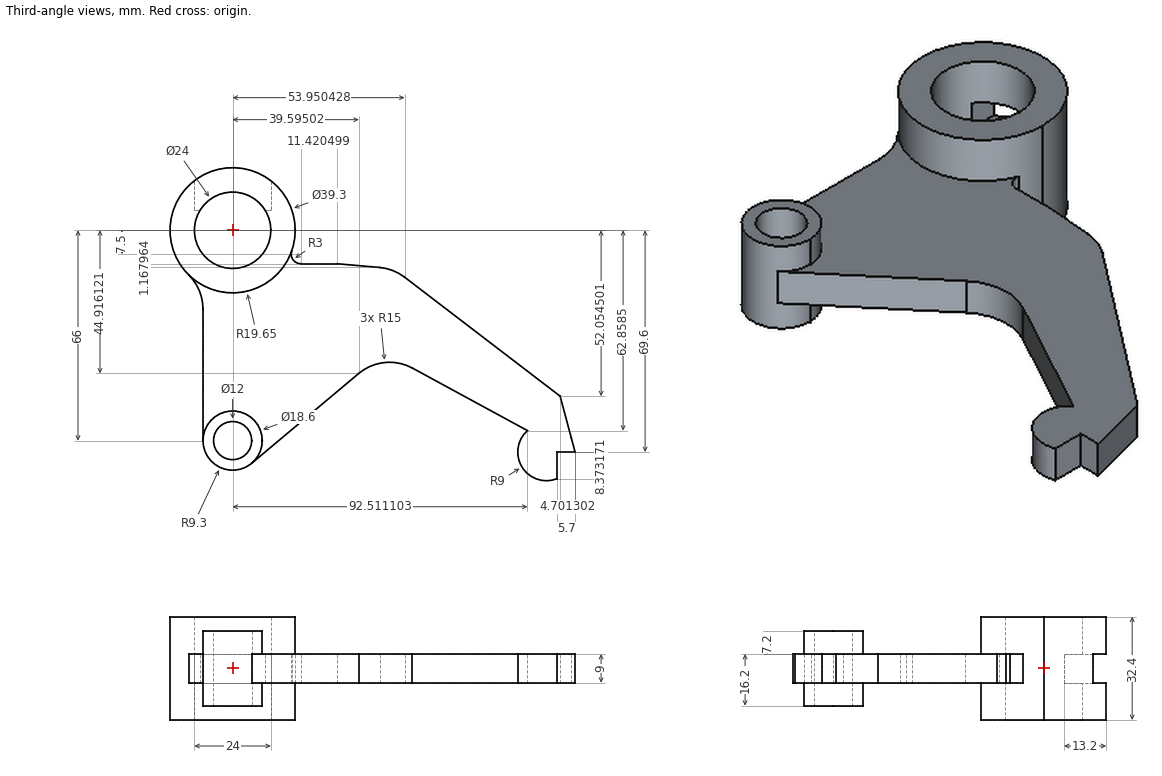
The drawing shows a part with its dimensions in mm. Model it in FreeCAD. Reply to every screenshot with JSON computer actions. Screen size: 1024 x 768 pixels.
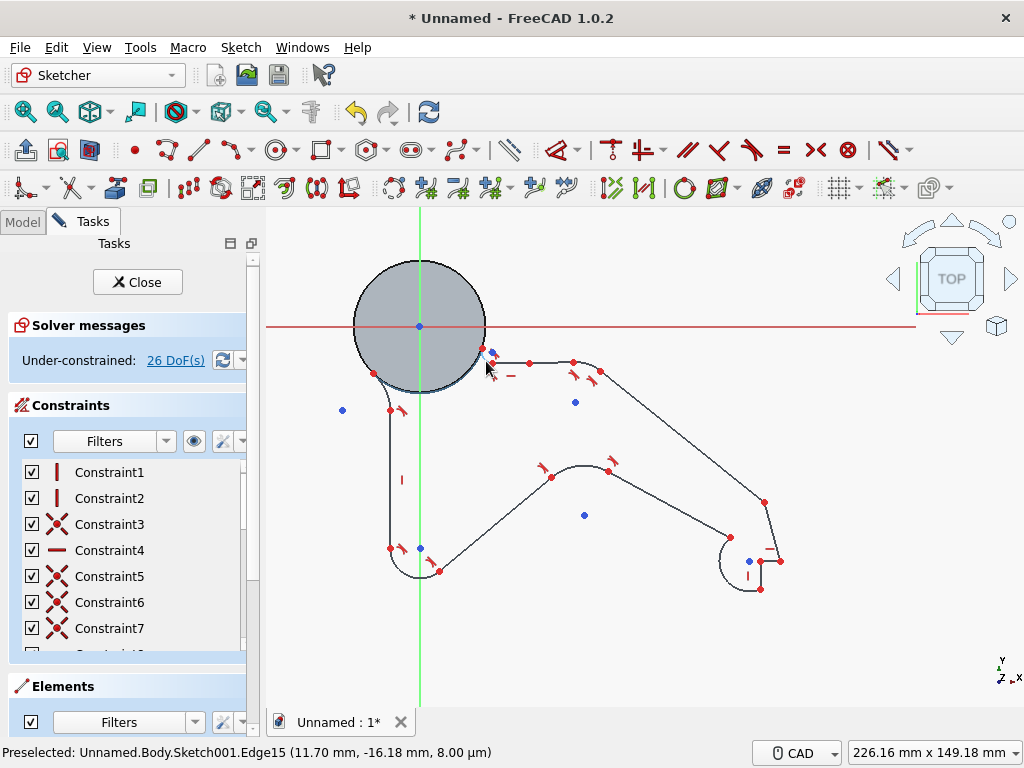
{"action": "left_click", "coordinate": [389, 398]}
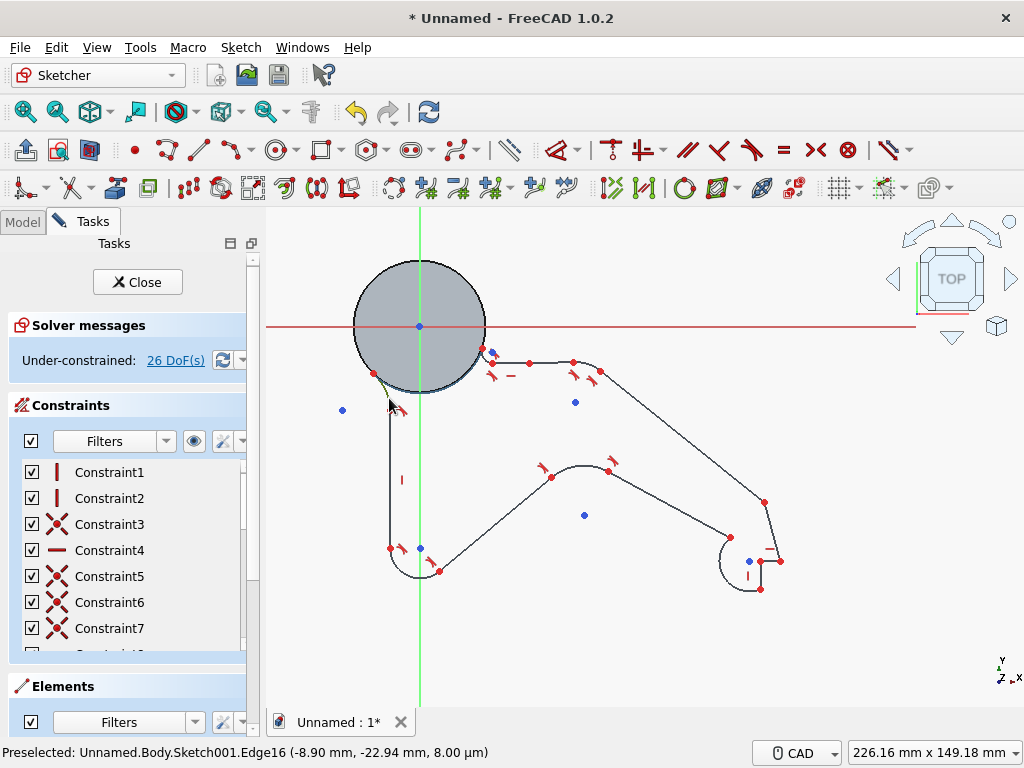
{"action": "key", "text": "t"}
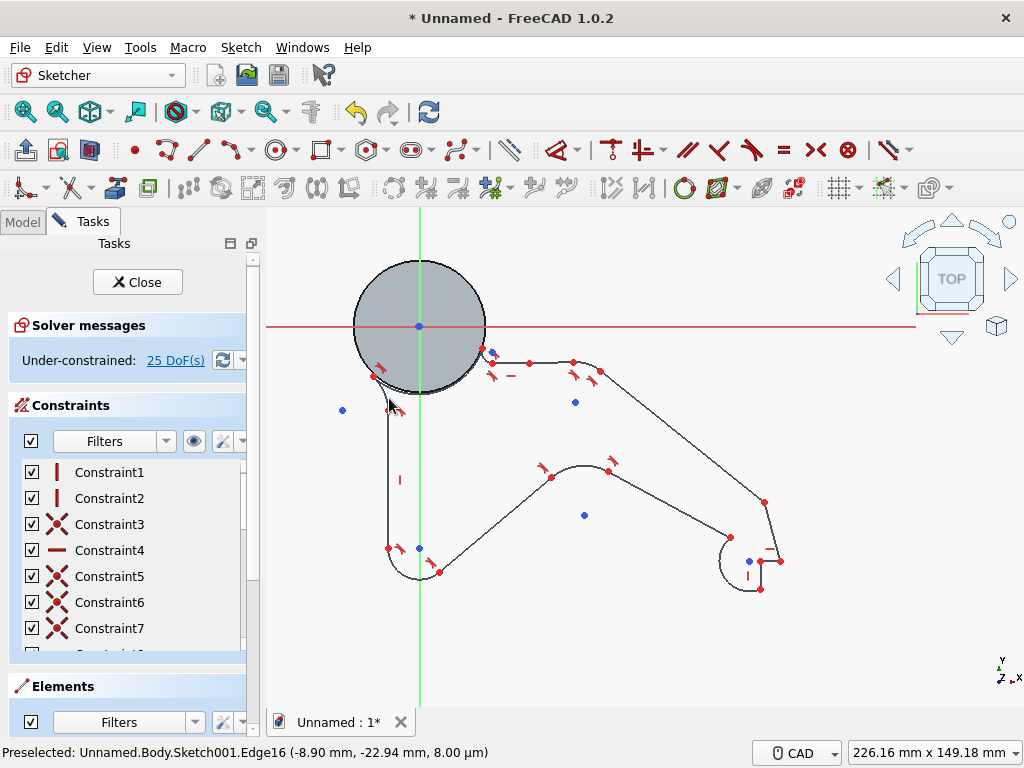
{"action": "scroll", "coordinate": [419, 327], "scroll_direction": "up", "scroll_amount": 7}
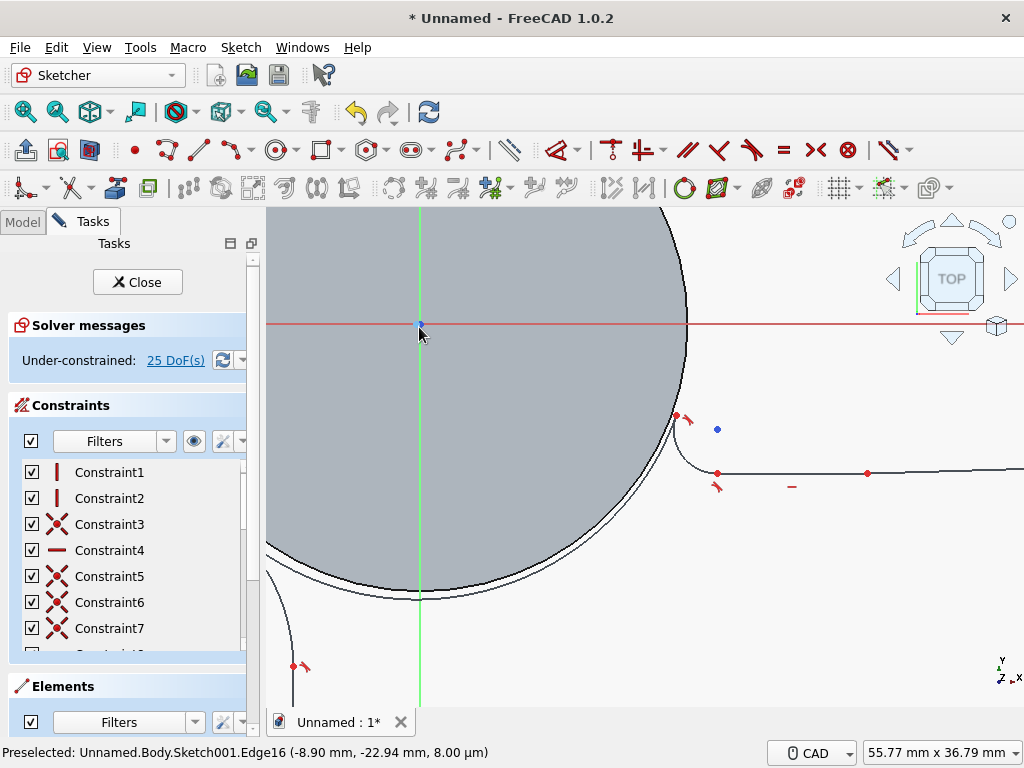
{"action": "left_click_drag", "start_coordinate": [407, 314], "coordinate": [430, 334]}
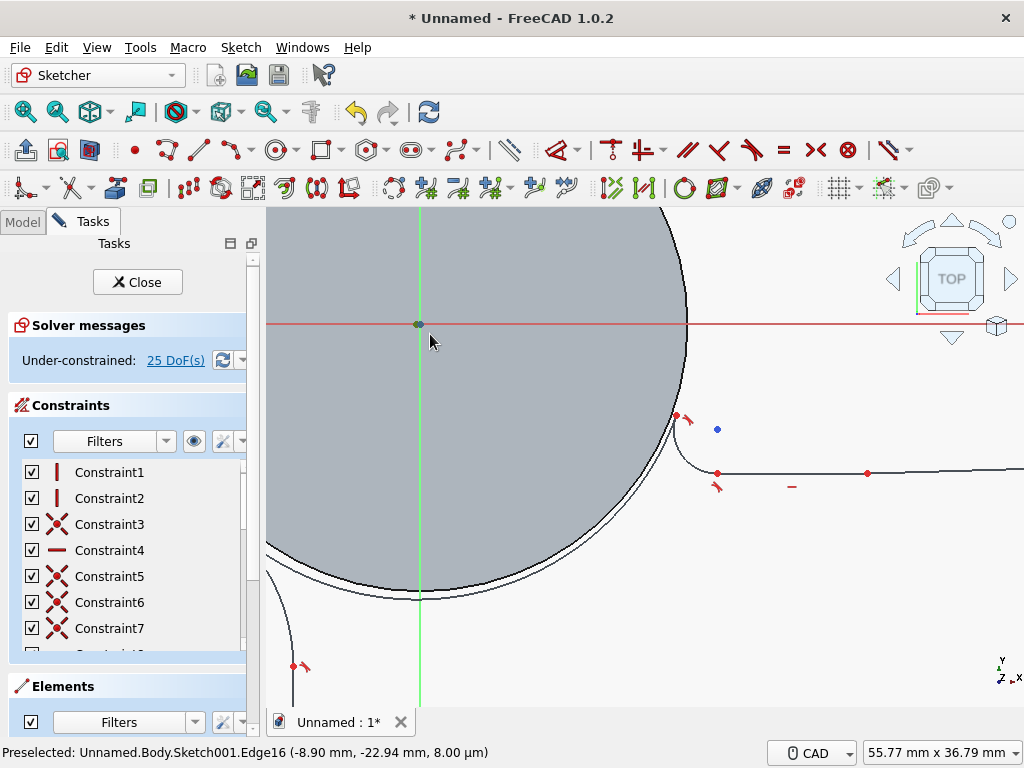
{"action": "key", "text": "c"}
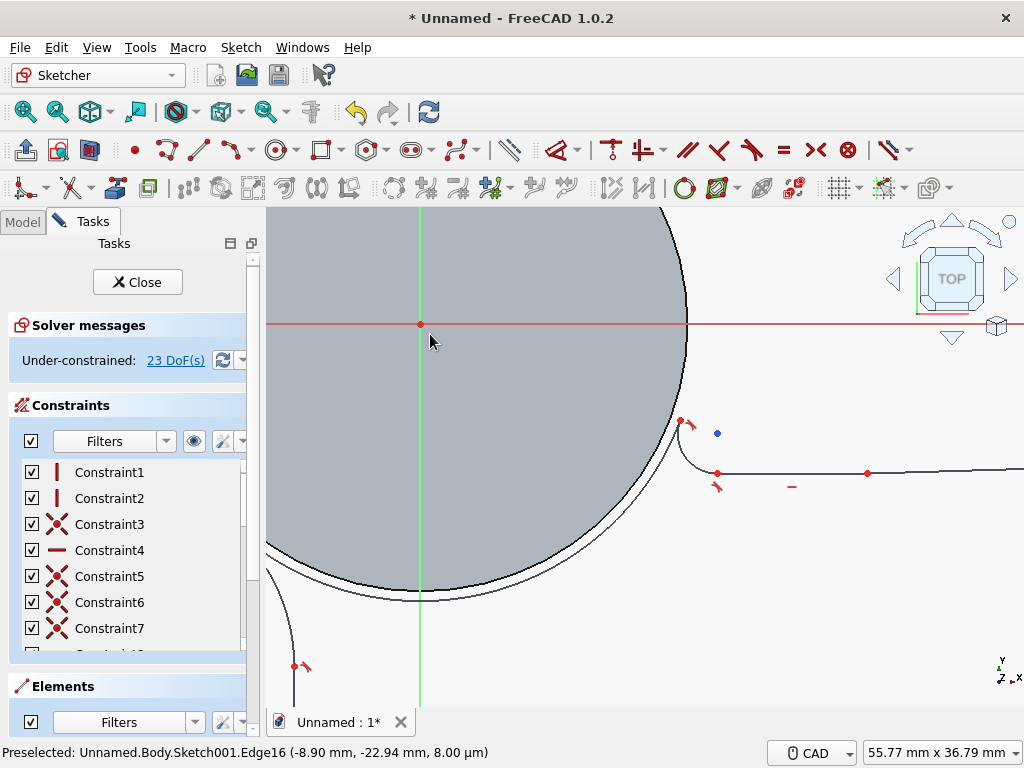
{"action": "scroll", "coordinate": [419, 327], "scroll_direction": "down", "scroll_amount": 7}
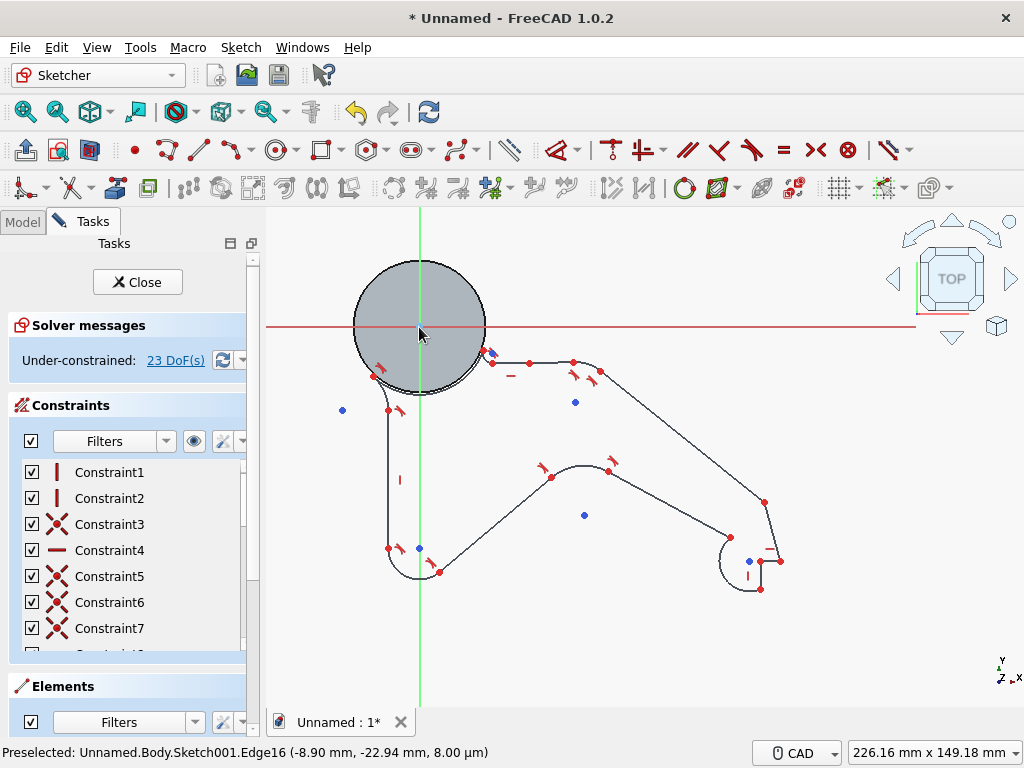
{"action": "left_click", "coordinate": [591, 466]}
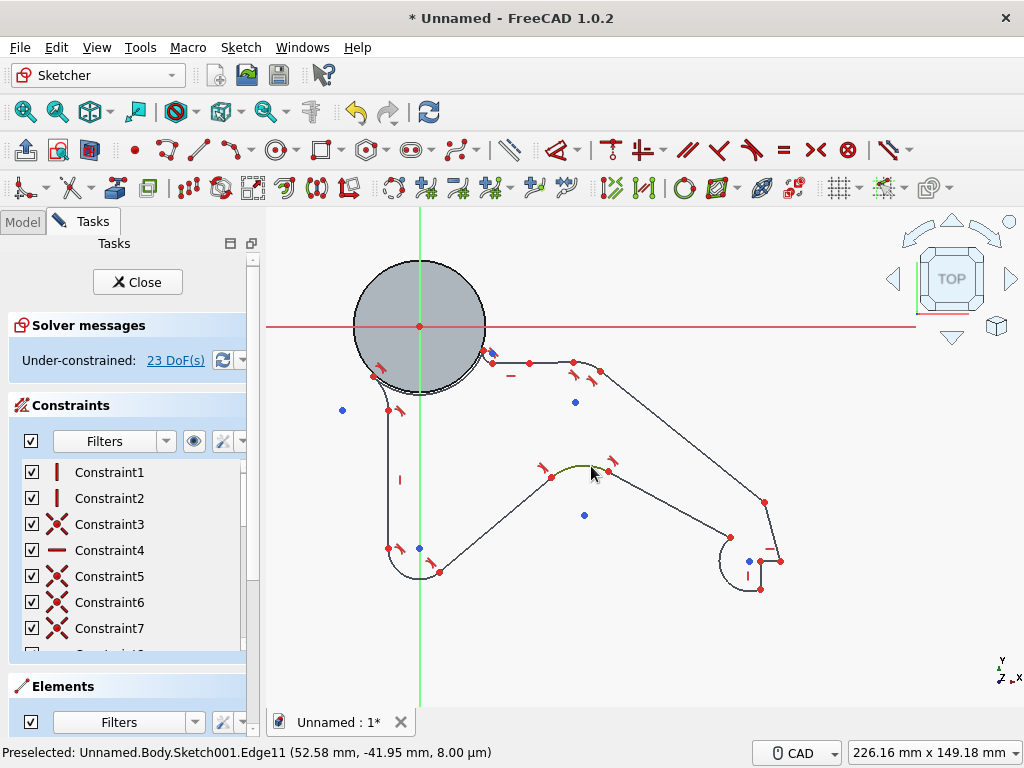
{"action": "left_click", "coordinate": [588, 364]}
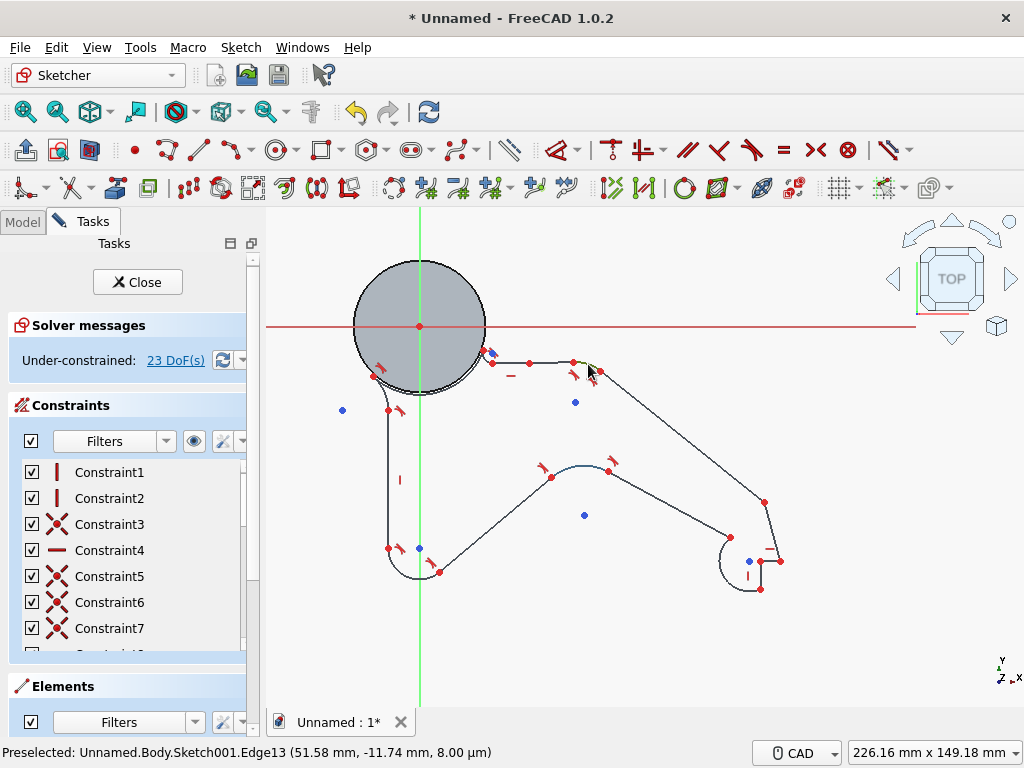
{"action": "left_click", "coordinate": [387, 400]}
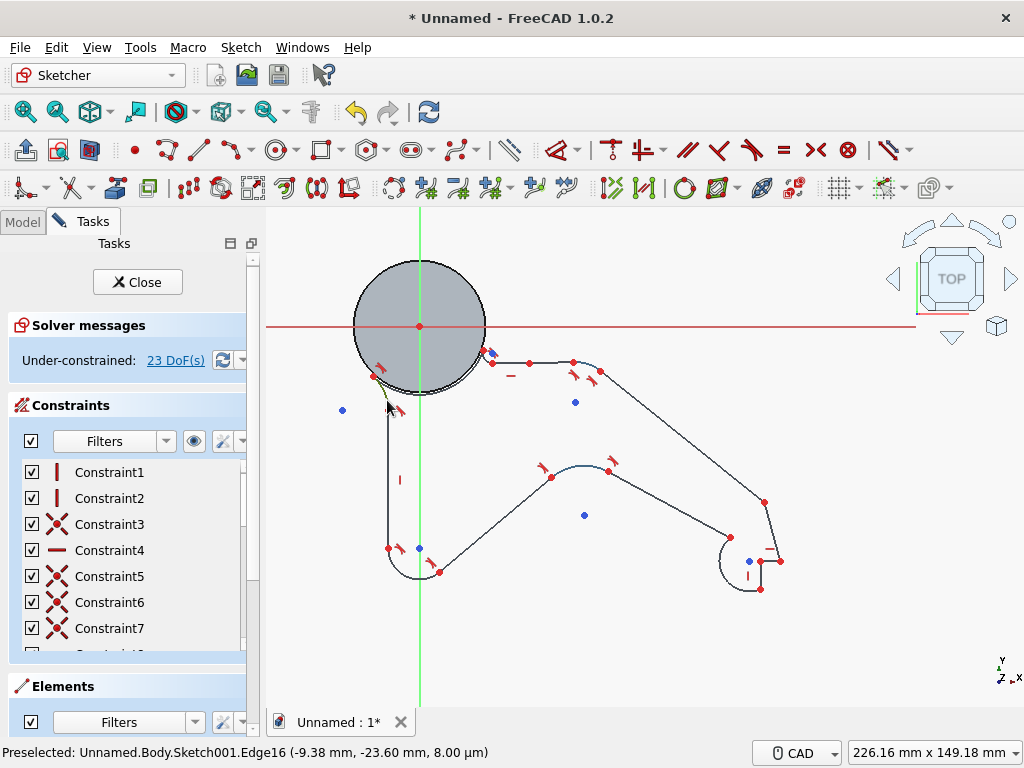
{"action": "key", "text": "e"}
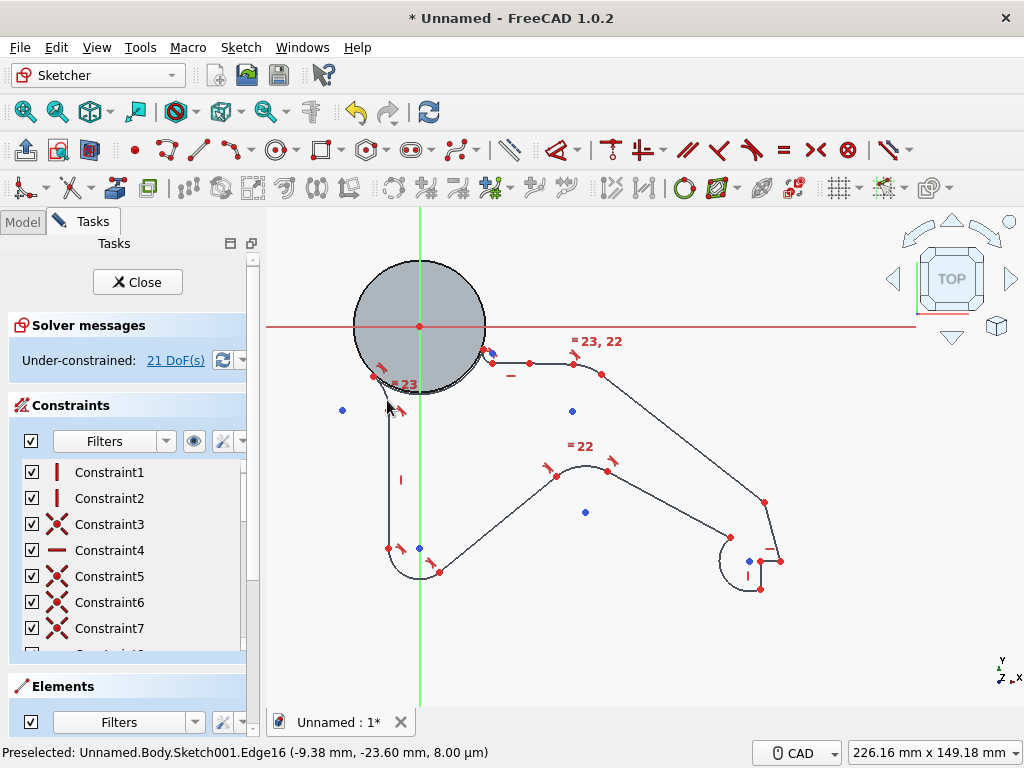
{"action": "left_click", "coordinate": [420, 548]}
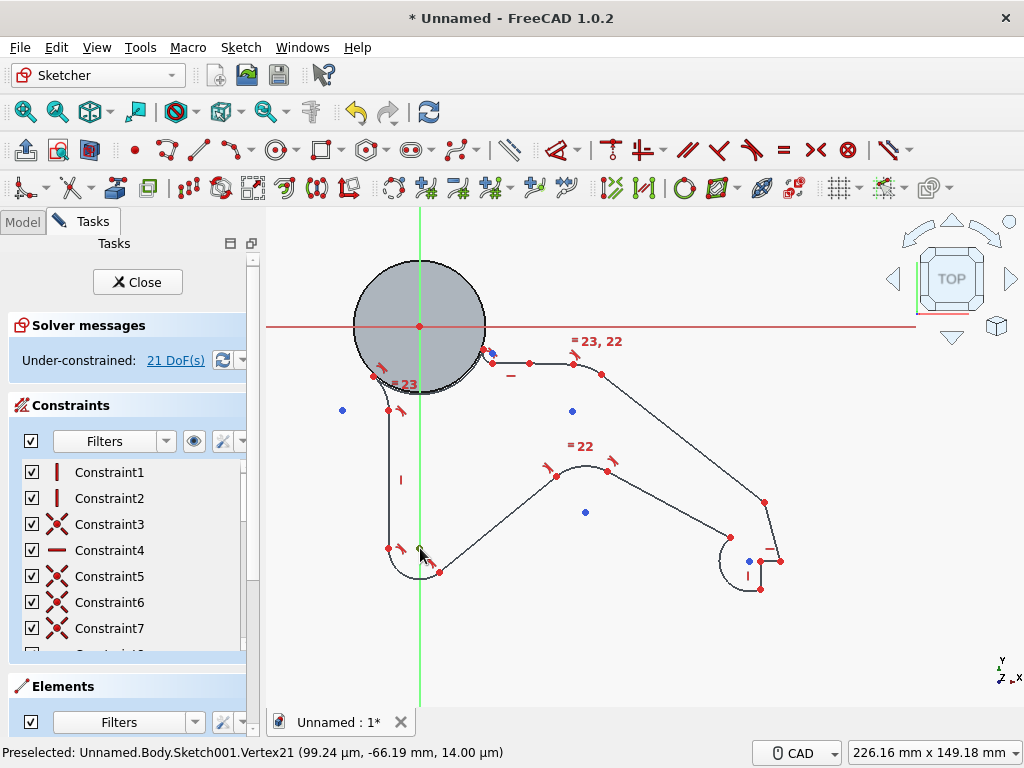
{"action": "left_click", "coordinate": [420, 647]}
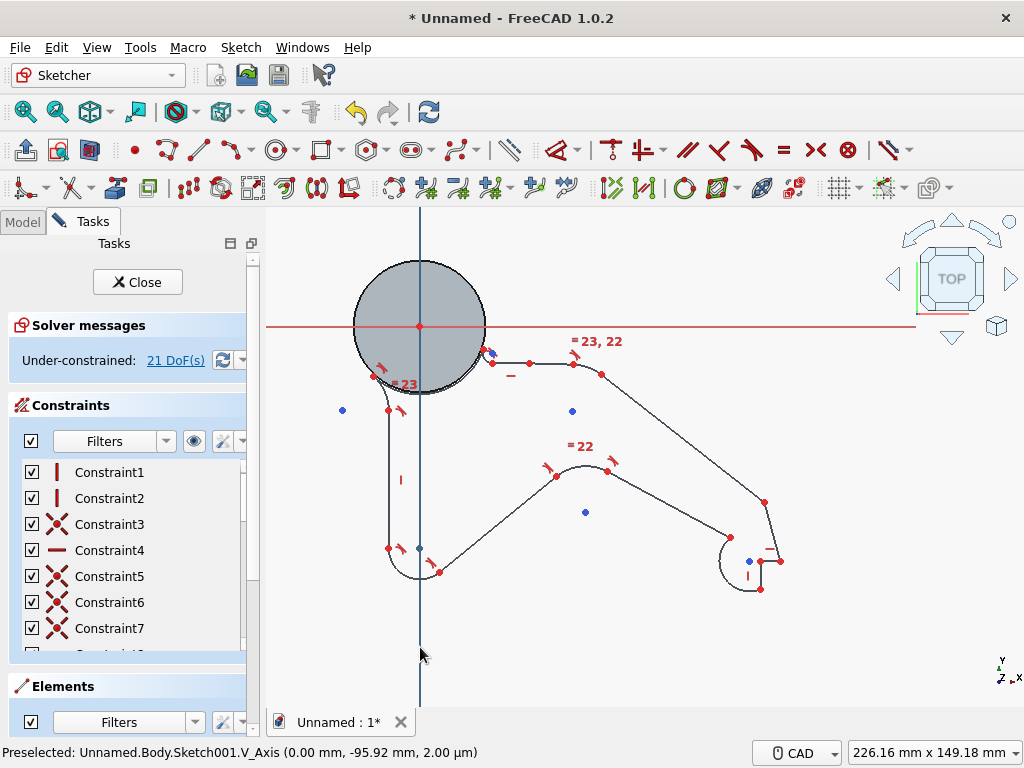
{"action": "key", "text": "c"}